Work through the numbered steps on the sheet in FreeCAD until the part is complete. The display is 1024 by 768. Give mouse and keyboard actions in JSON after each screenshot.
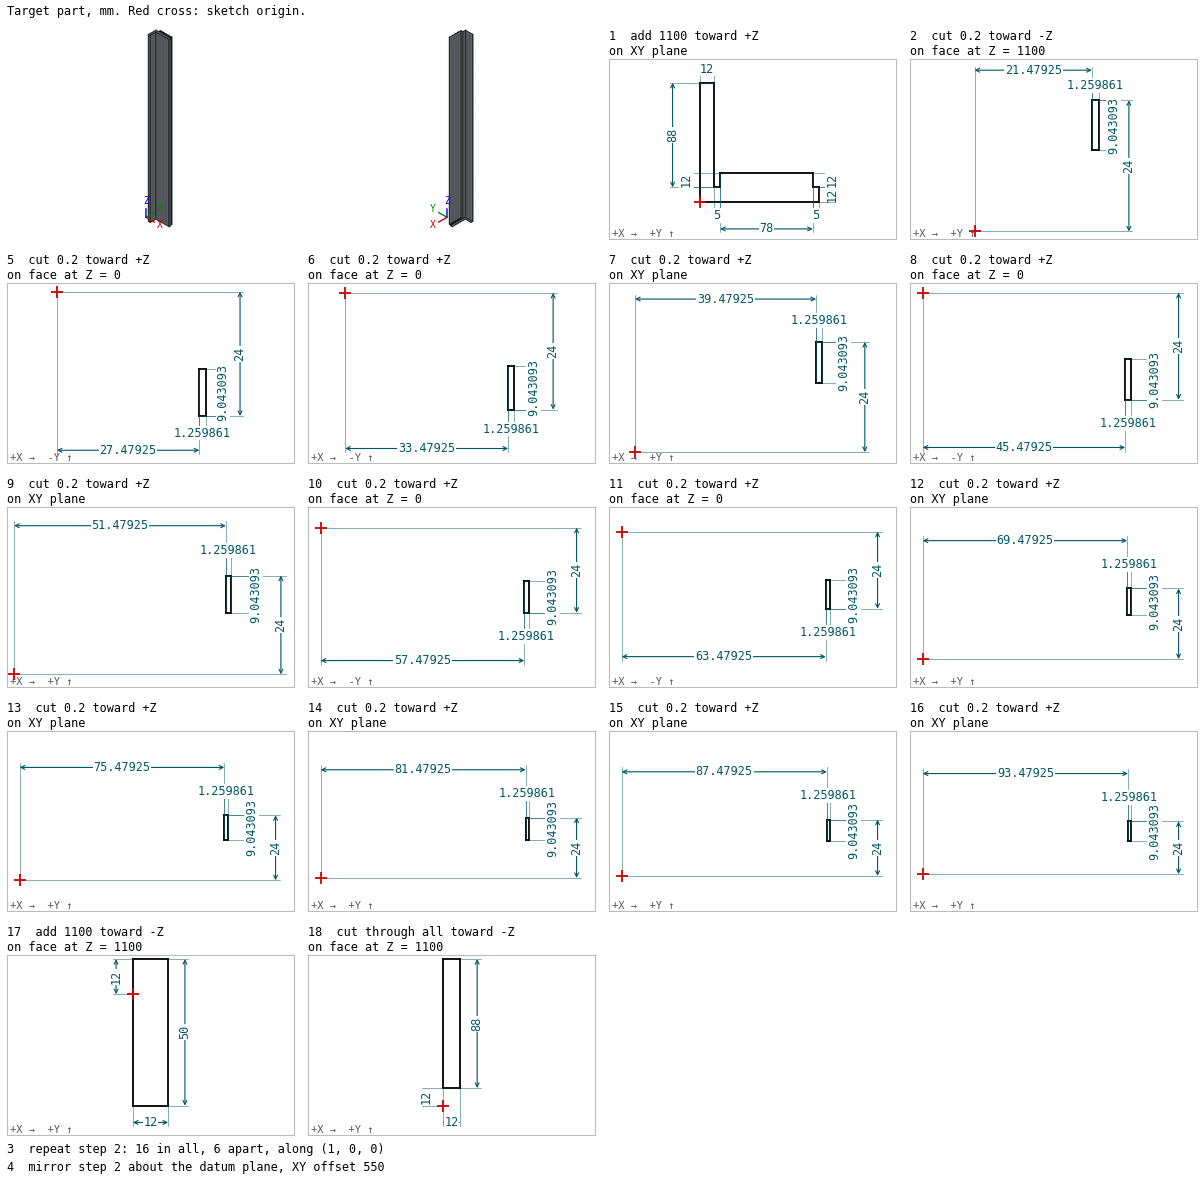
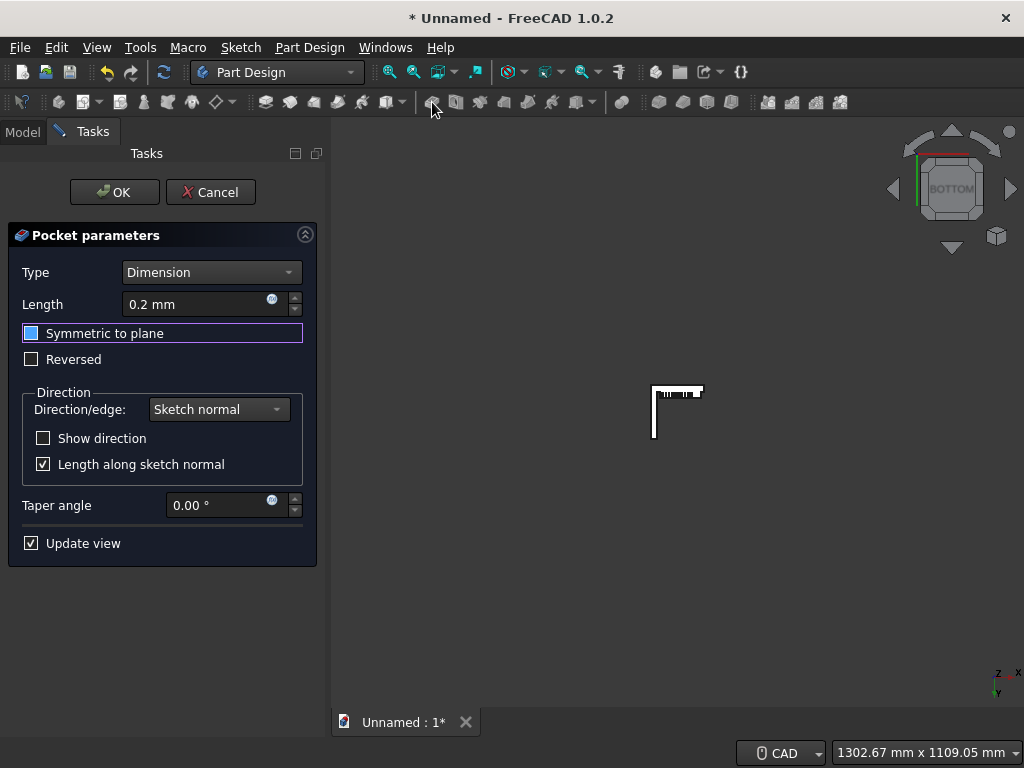
{"action": "left_click", "coordinate": [30, 359]}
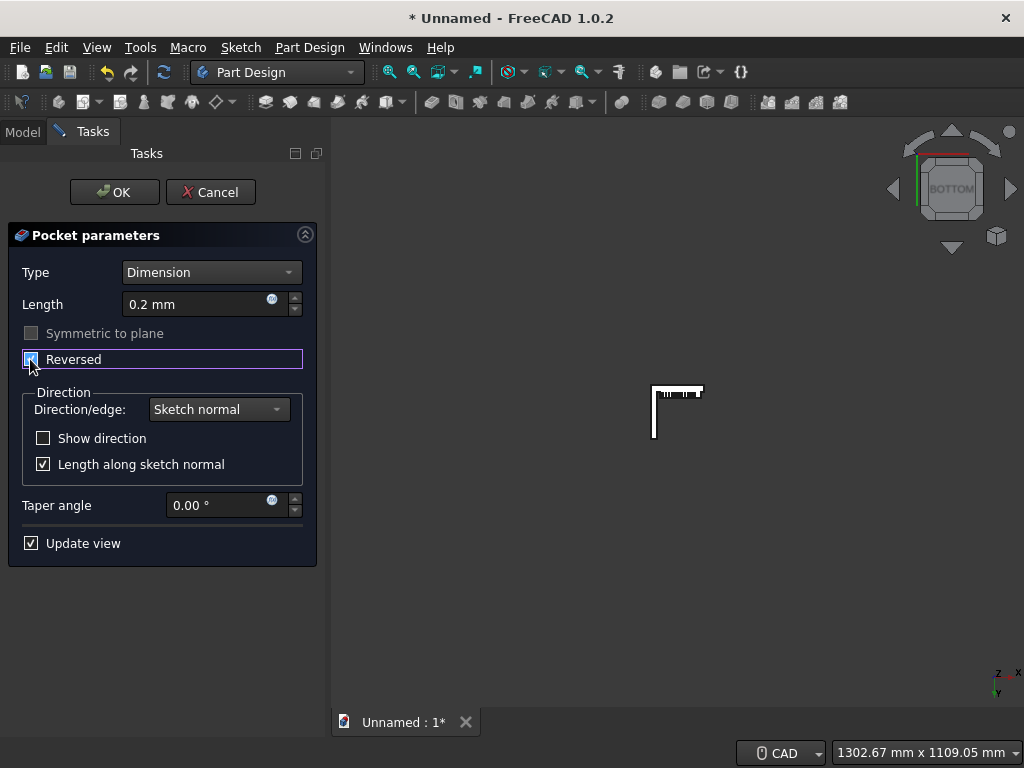
{"action": "left_click", "coordinate": [115, 192]}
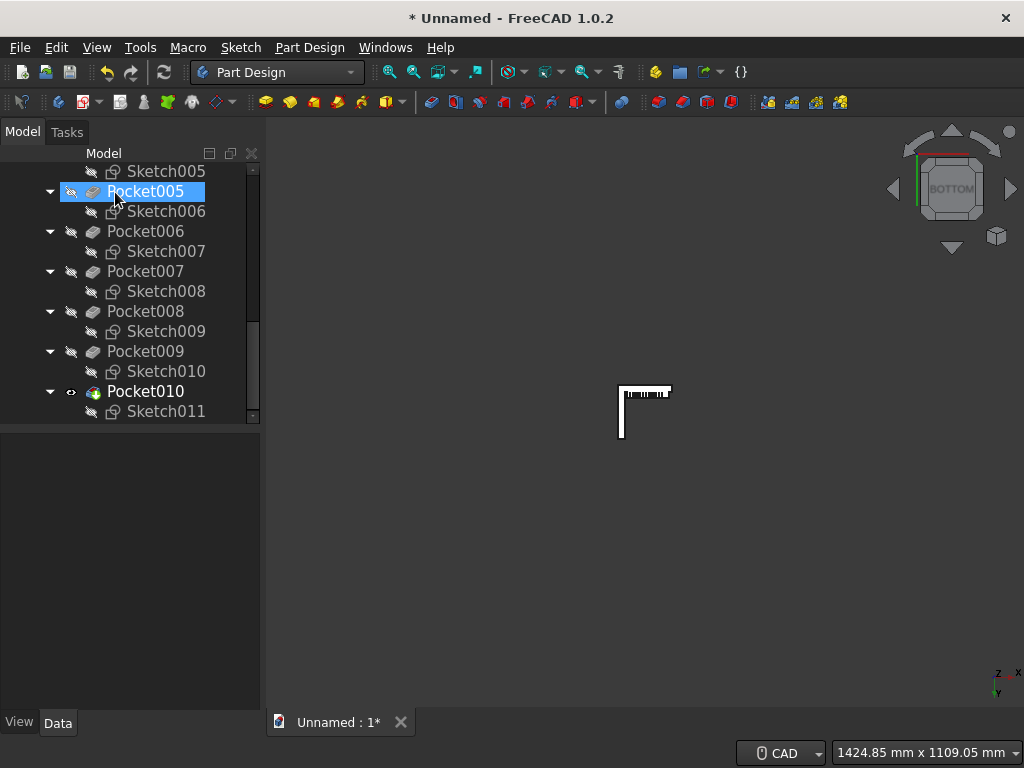
{"action": "left_click", "coordinate": [390, 72]}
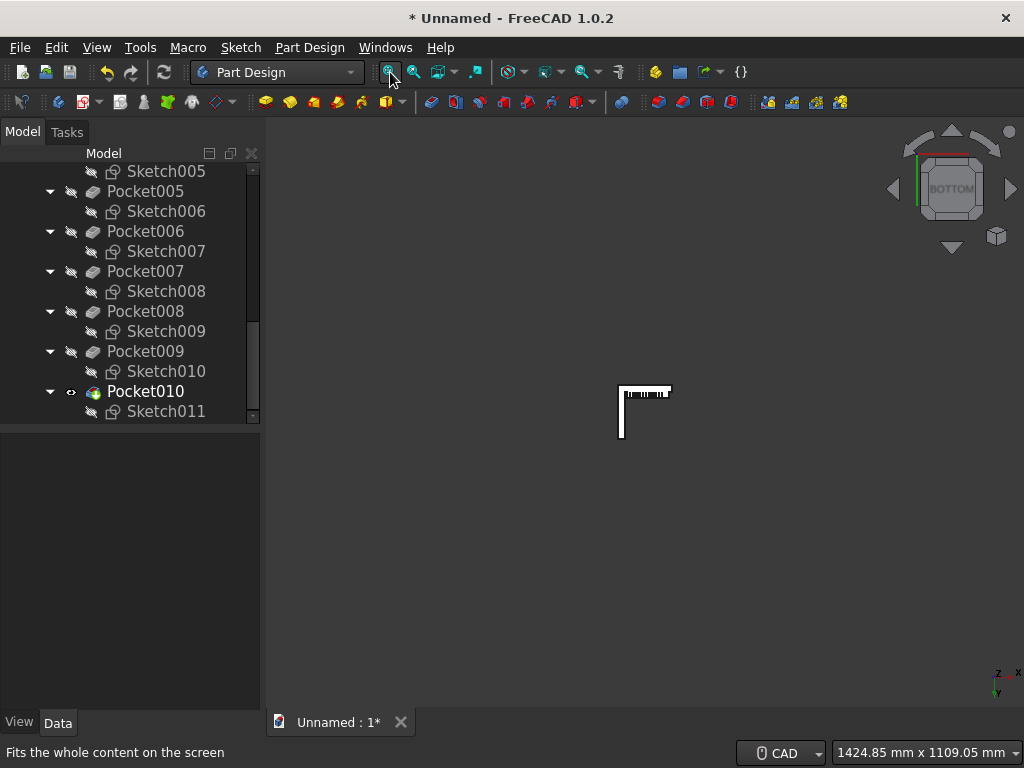
{"action": "left_click", "coordinate": [84, 102]}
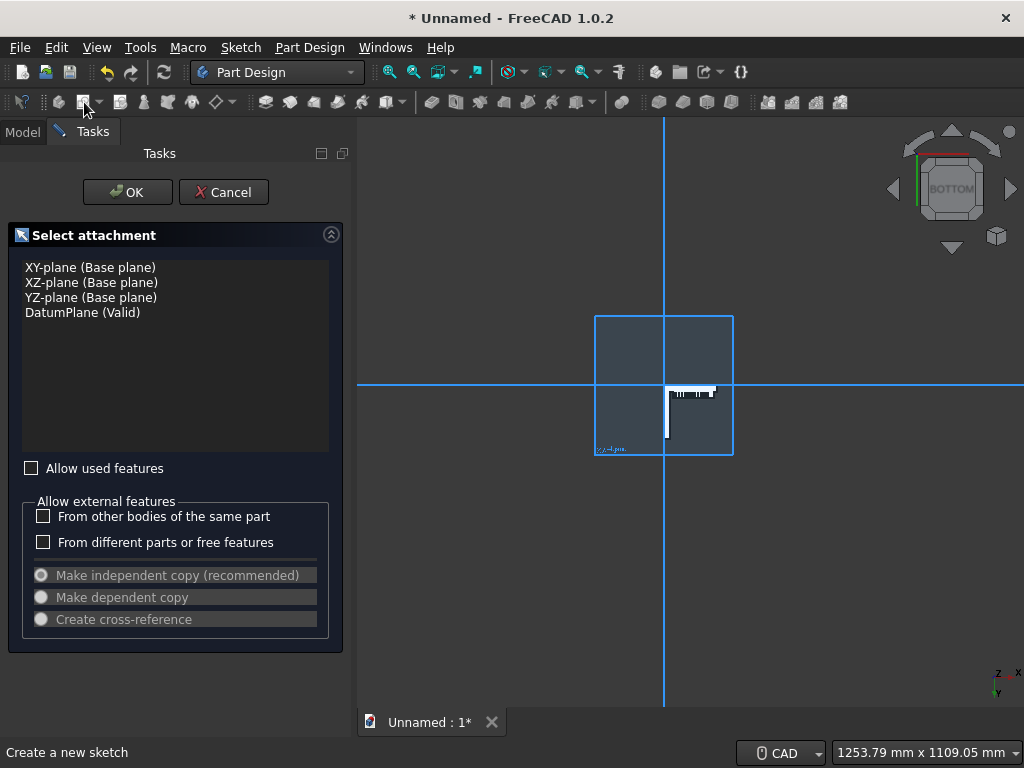
{"action": "left_click", "coordinate": [82, 268]}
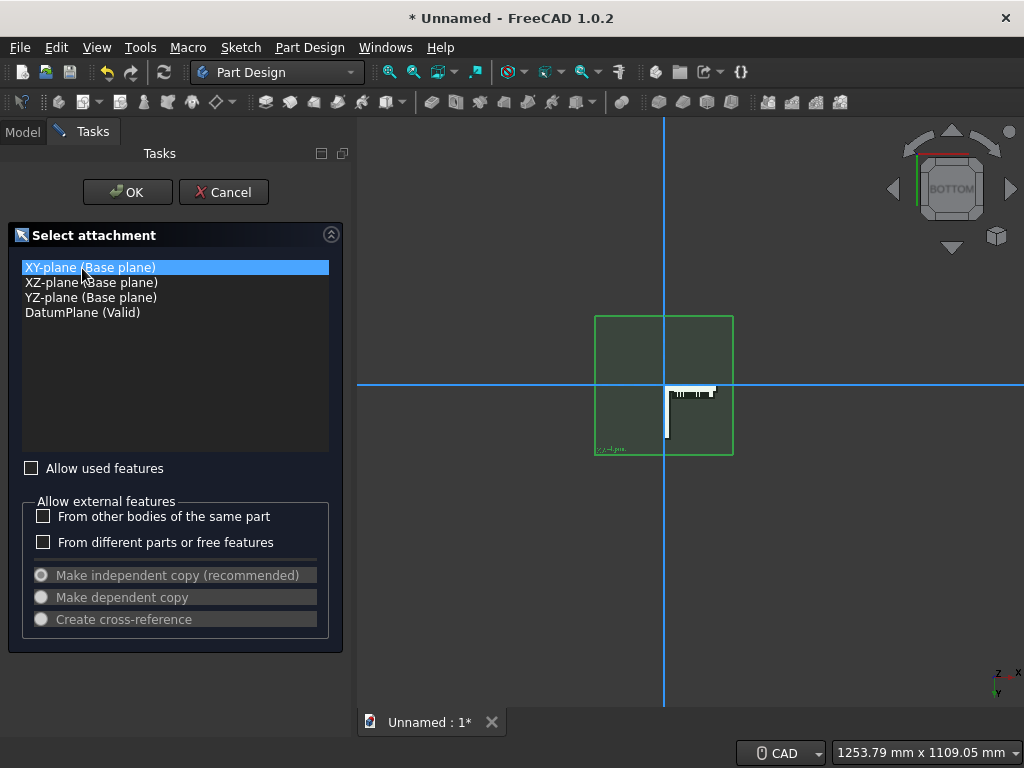
{"action": "left_click", "coordinate": [128, 192]}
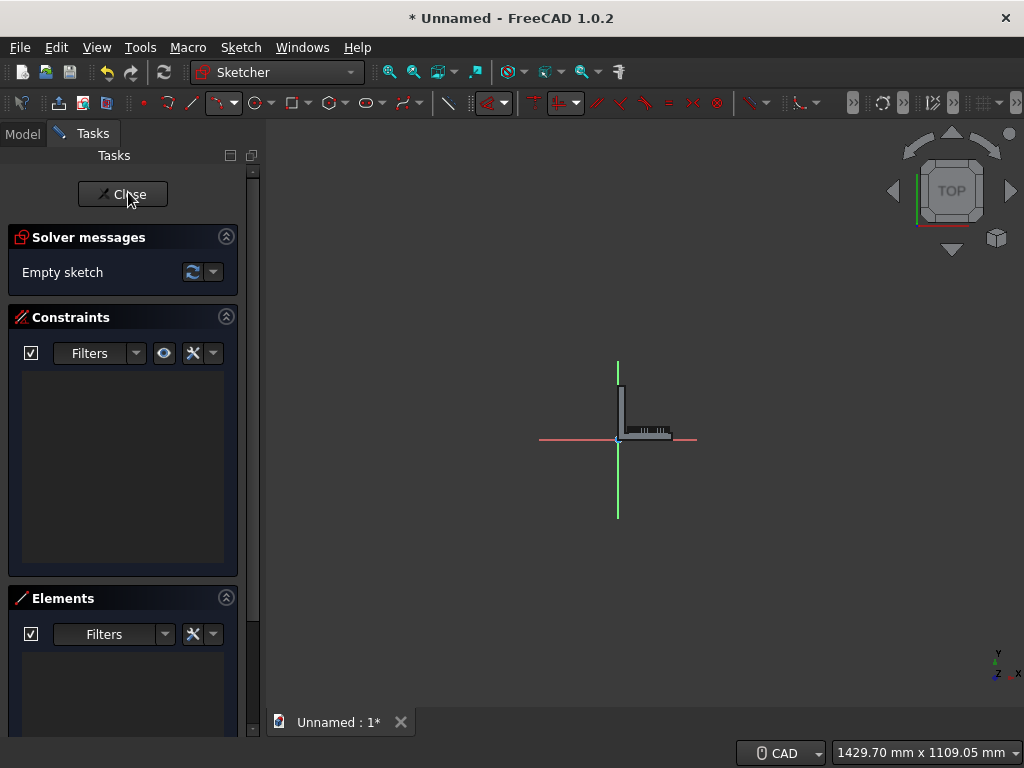
{"action": "left_click", "coordinate": [108, 104]}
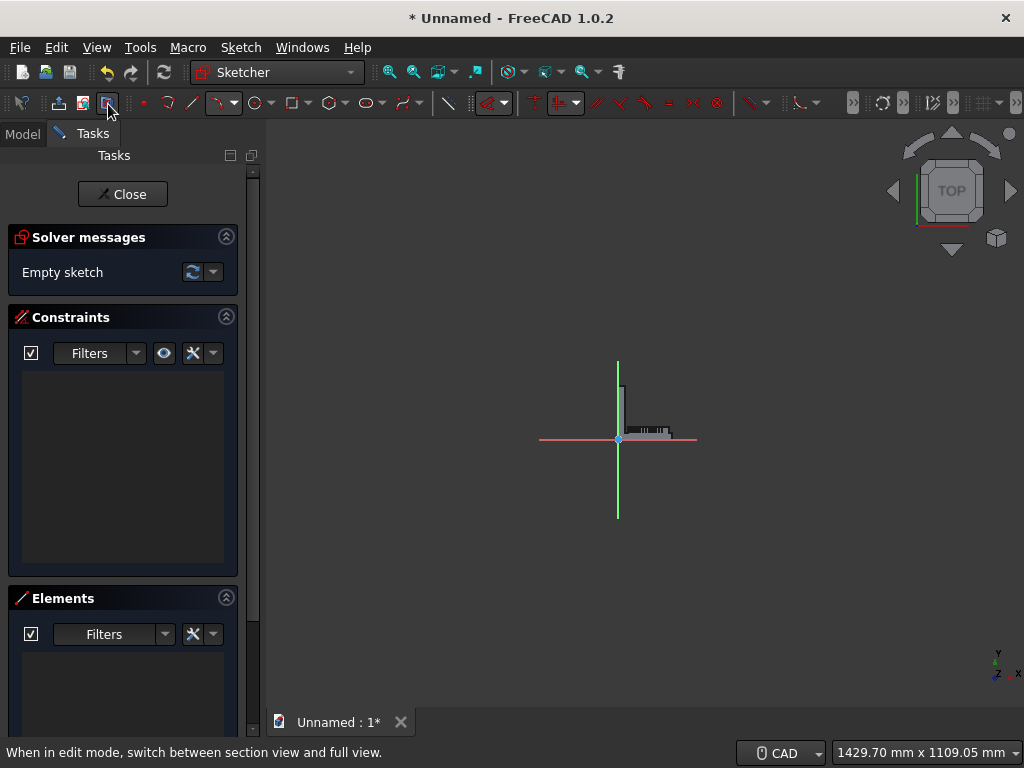
{"action": "scroll", "coordinate": [670, 430], "scroll_direction": "up", "scroll_amount": 15}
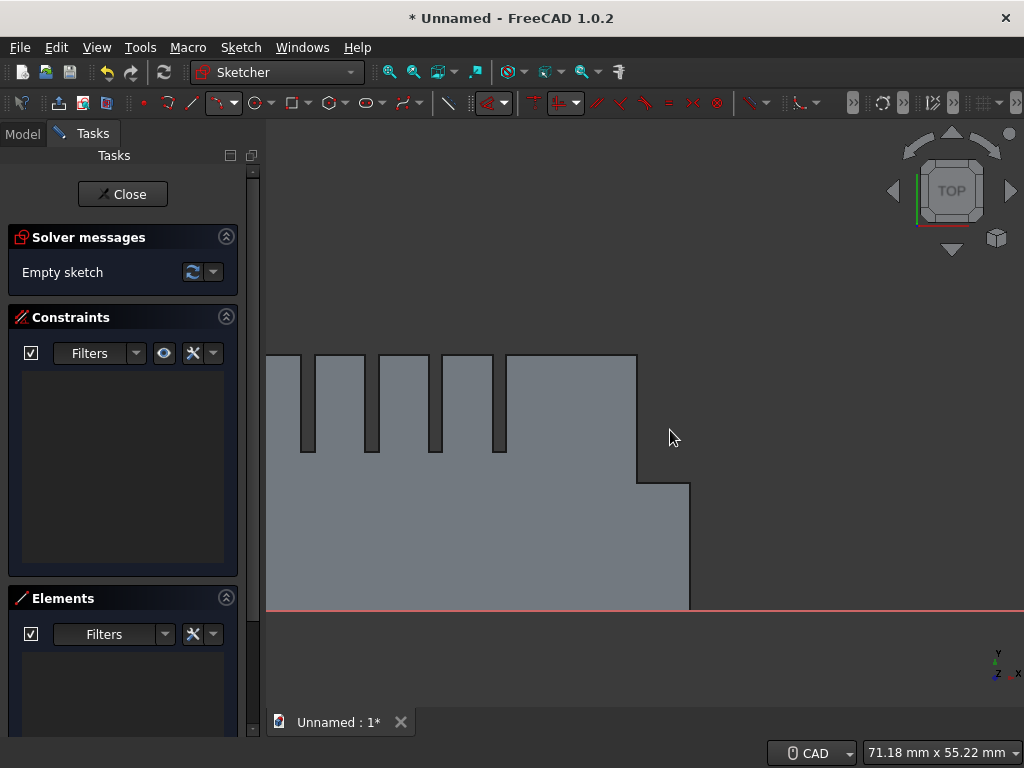
{"action": "scroll", "coordinate": [559, 400], "scroll_direction": "up", "scroll_amount": 7}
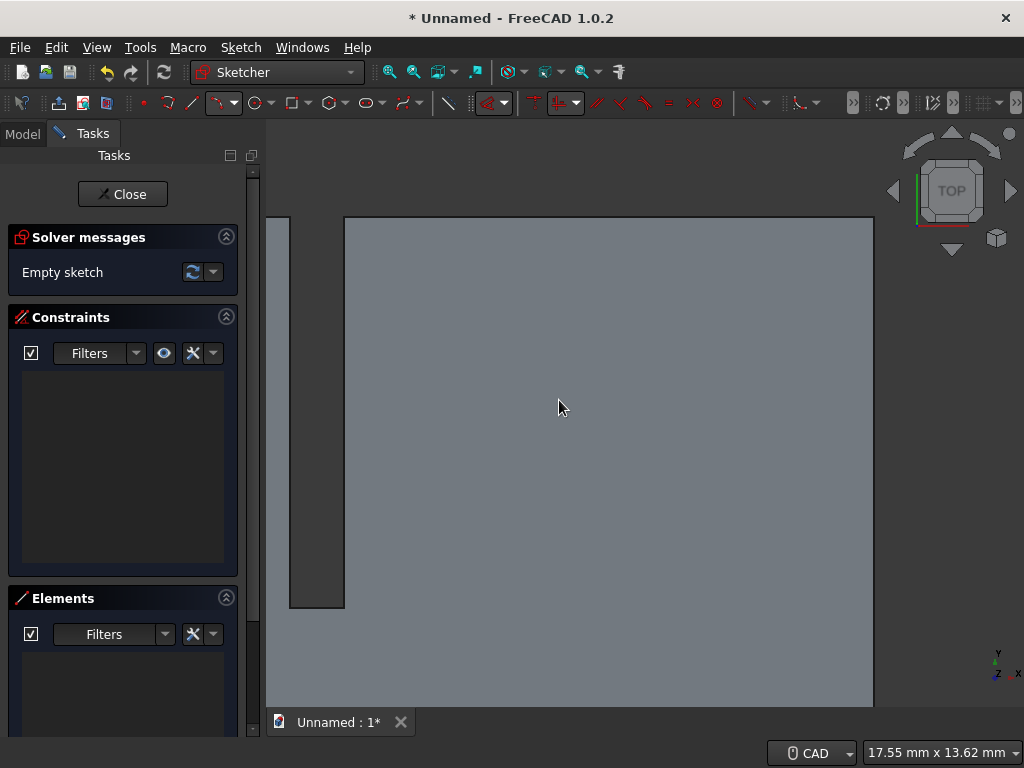
{"action": "key", "text": "g r"}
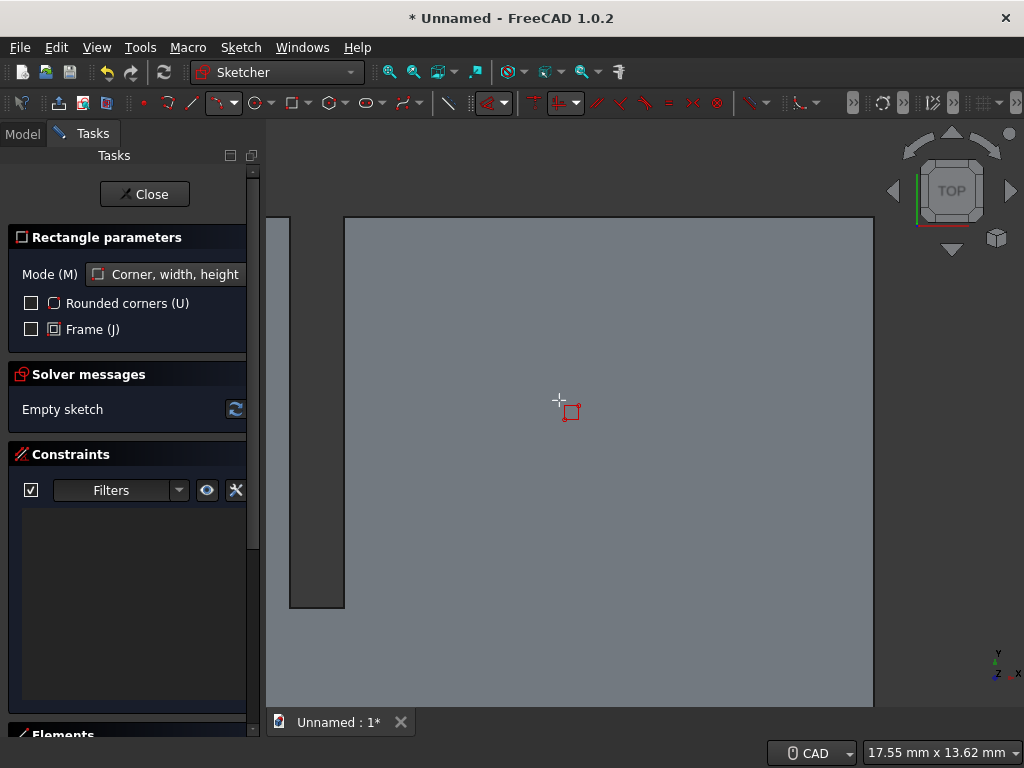
{"action": "left_click", "coordinate": [549, 217]}
{"action": "mouse_move", "coordinate": [603, 608]}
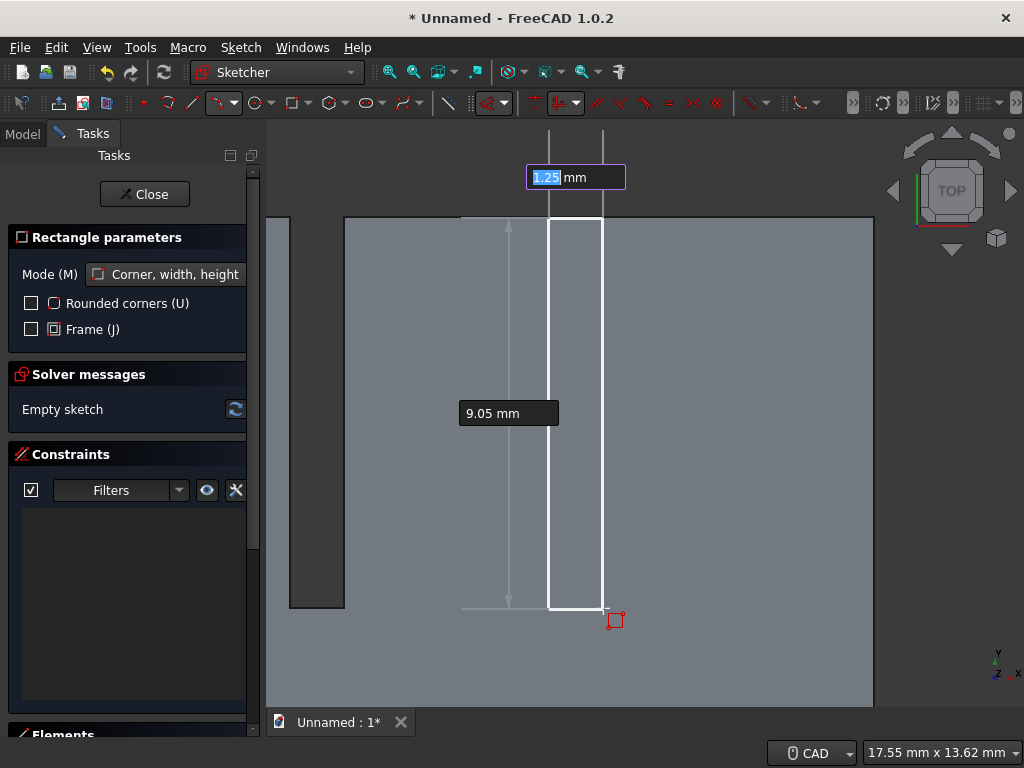
{"action": "type", "text": "1.259861"}
{"action": "key", "text": "Tab"}
{"action": "type", "text": "9.043093"}
{"action": "key", "text": "Return"}
{"action": "key", "text": "Escape"}